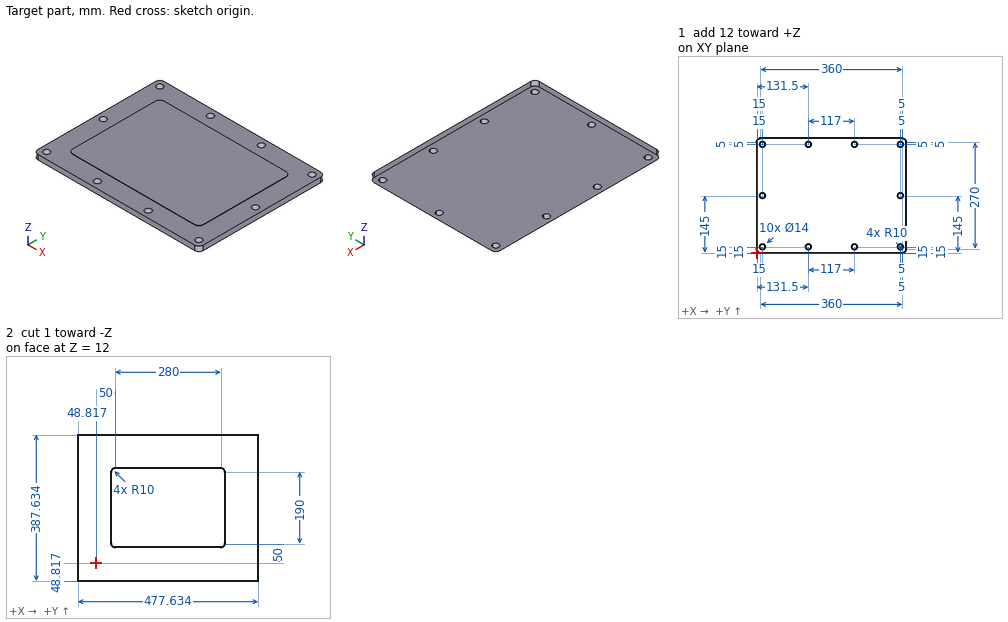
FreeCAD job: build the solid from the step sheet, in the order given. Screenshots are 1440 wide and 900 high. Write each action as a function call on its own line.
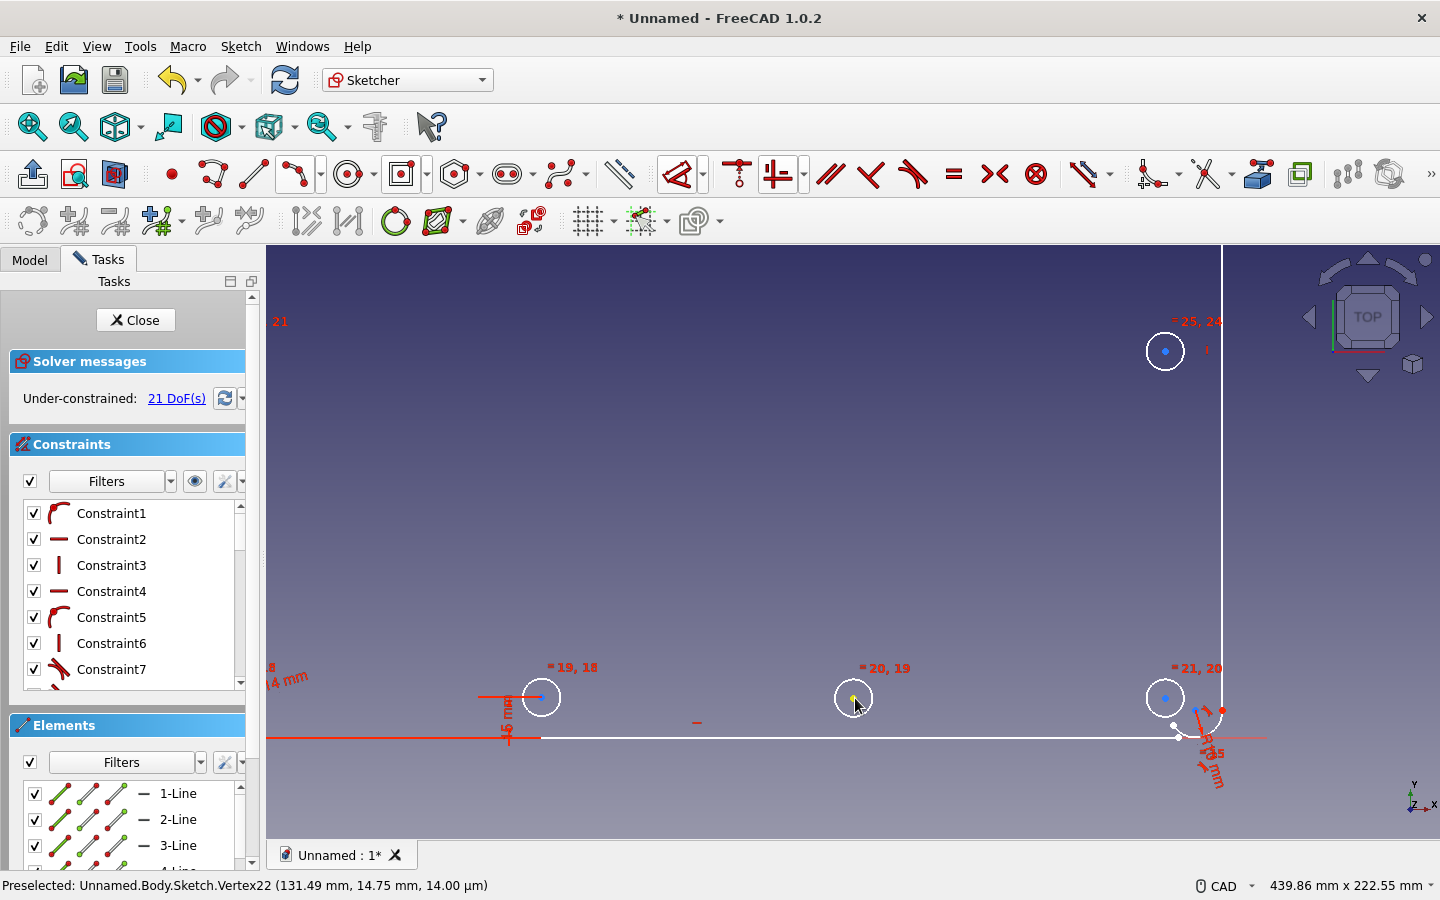
click(854, 698)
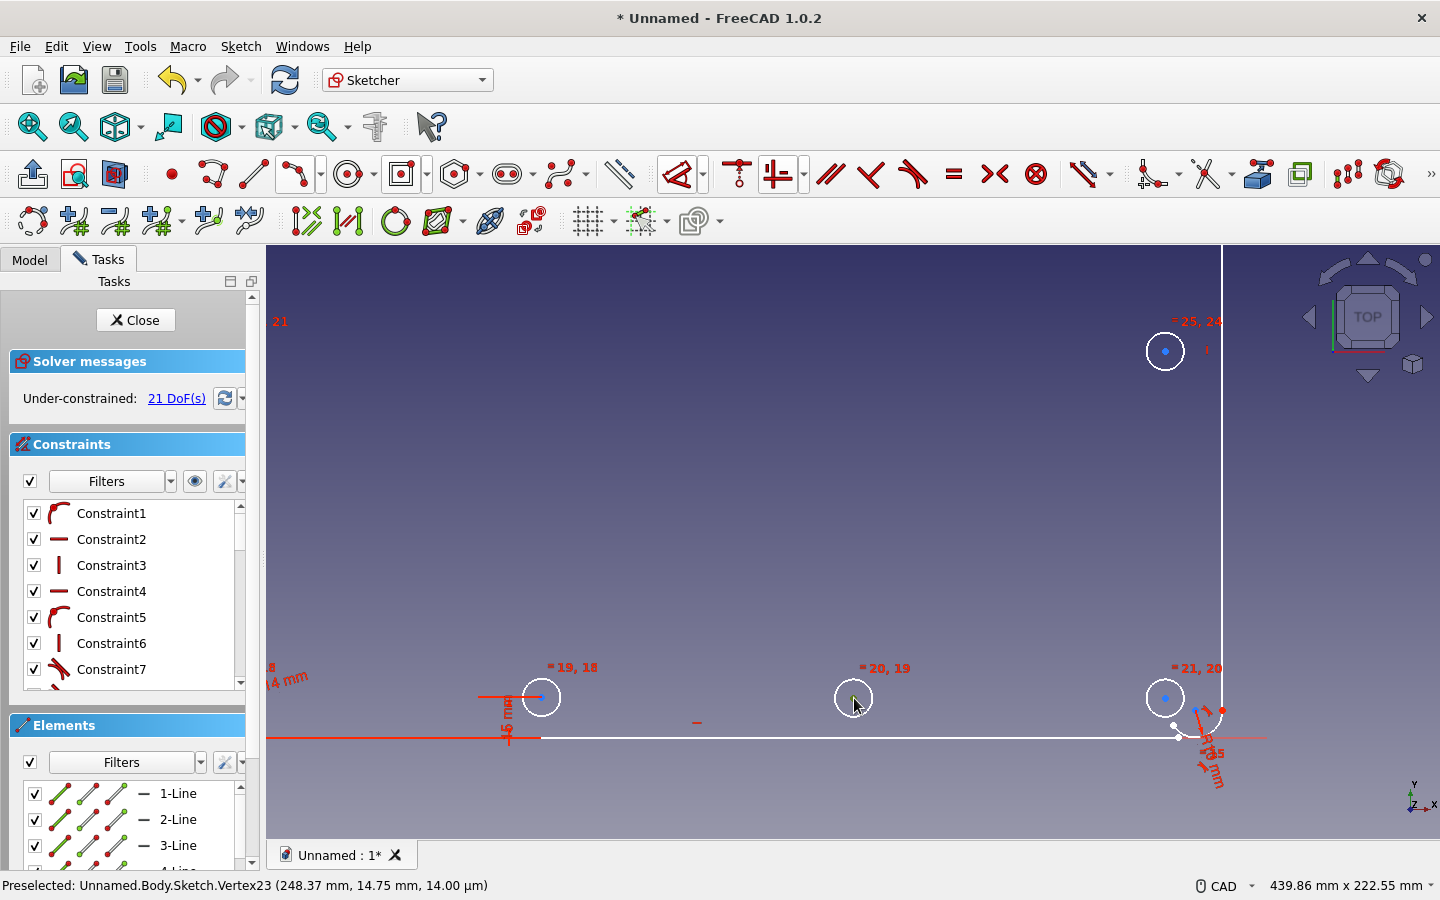
click(702, 174)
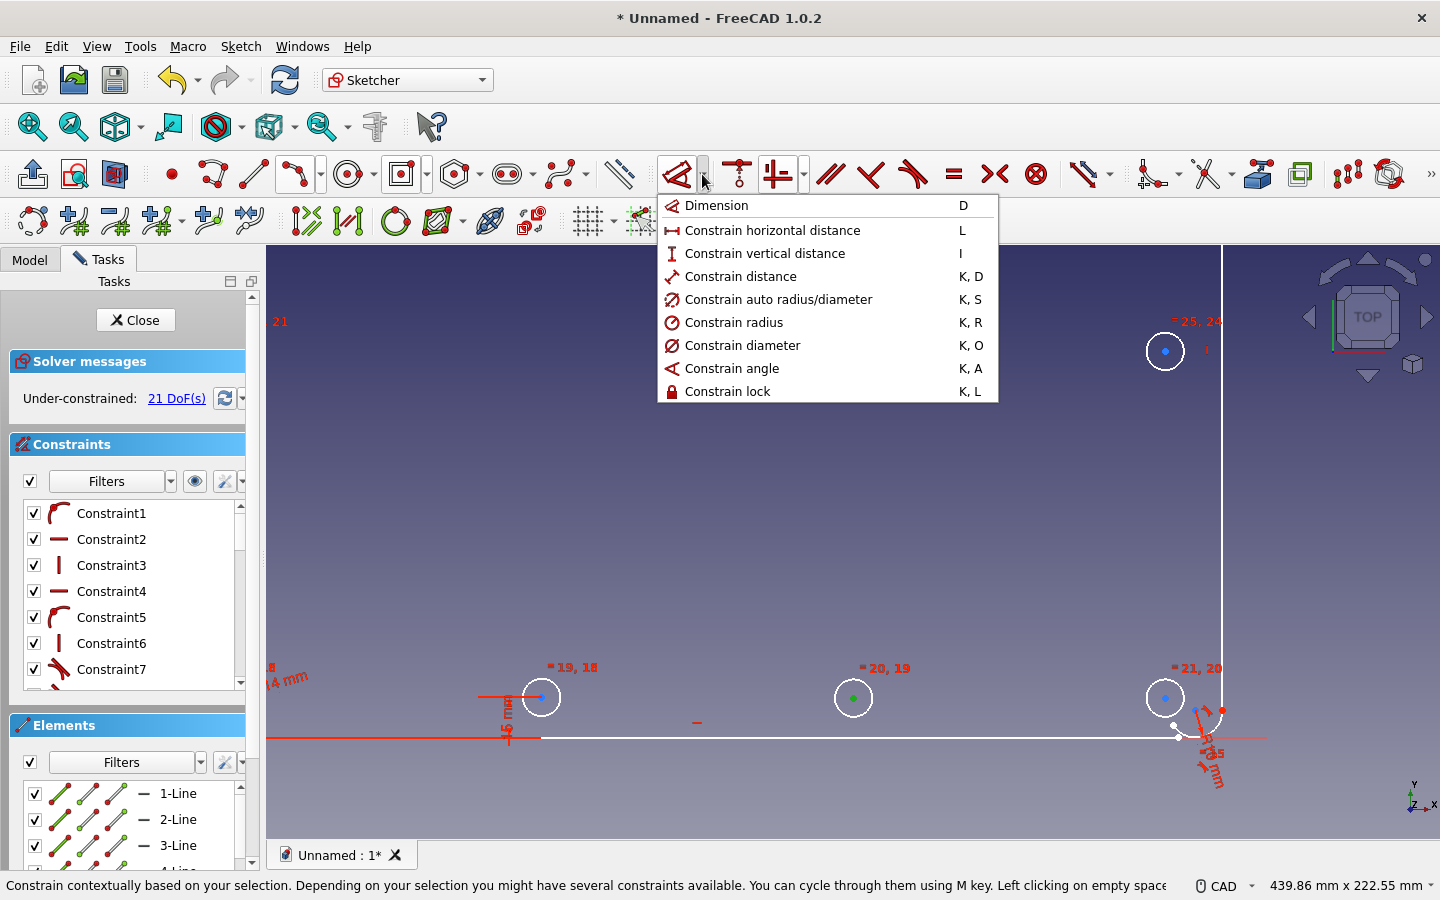
click(828, 254)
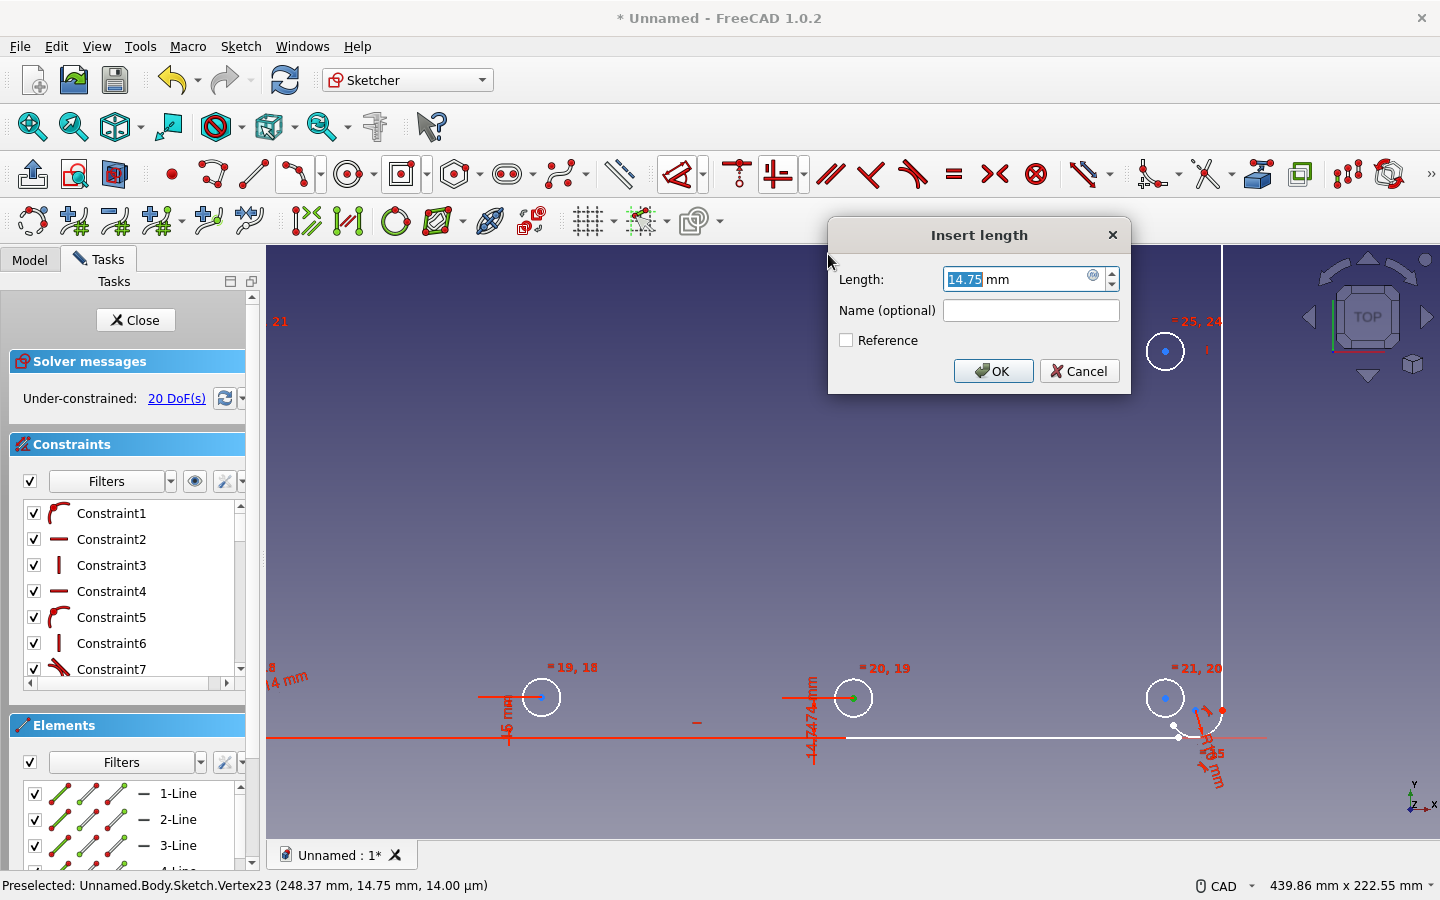
text(15)
key(Return)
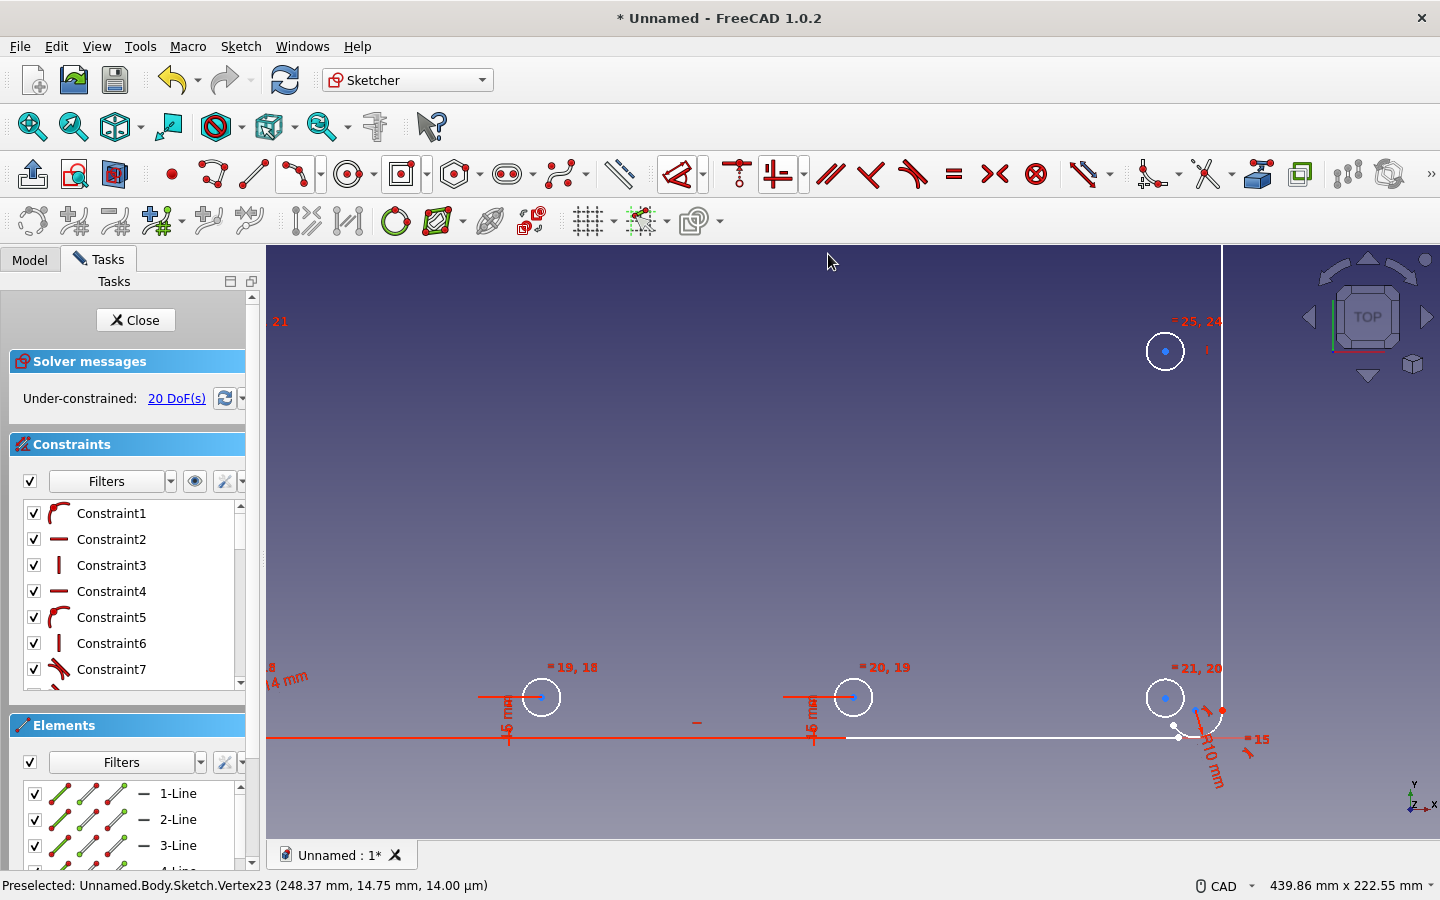
click(1165, 698)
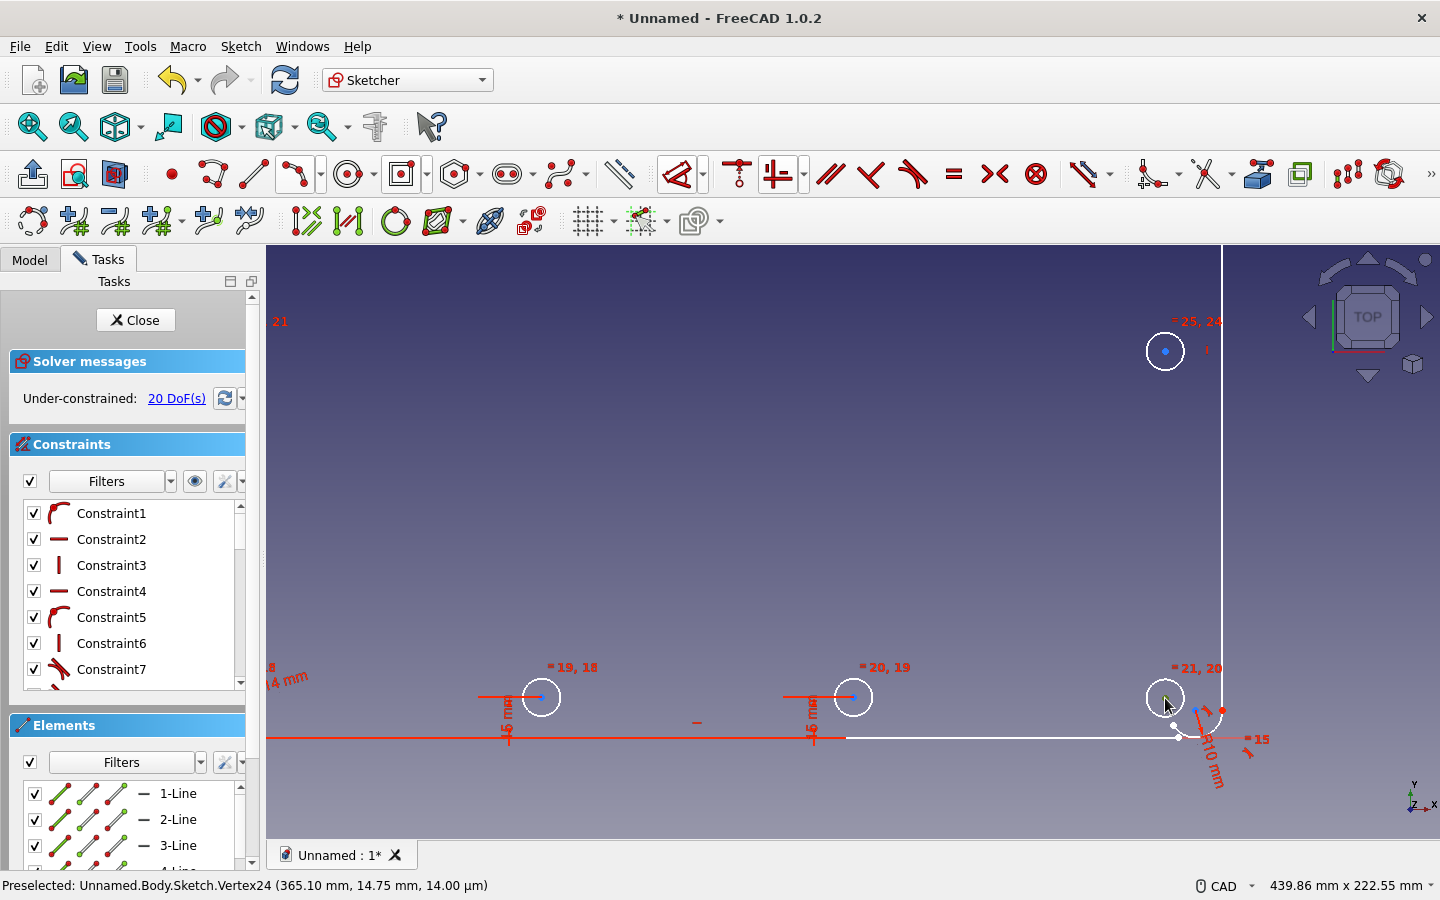
click(702, 174)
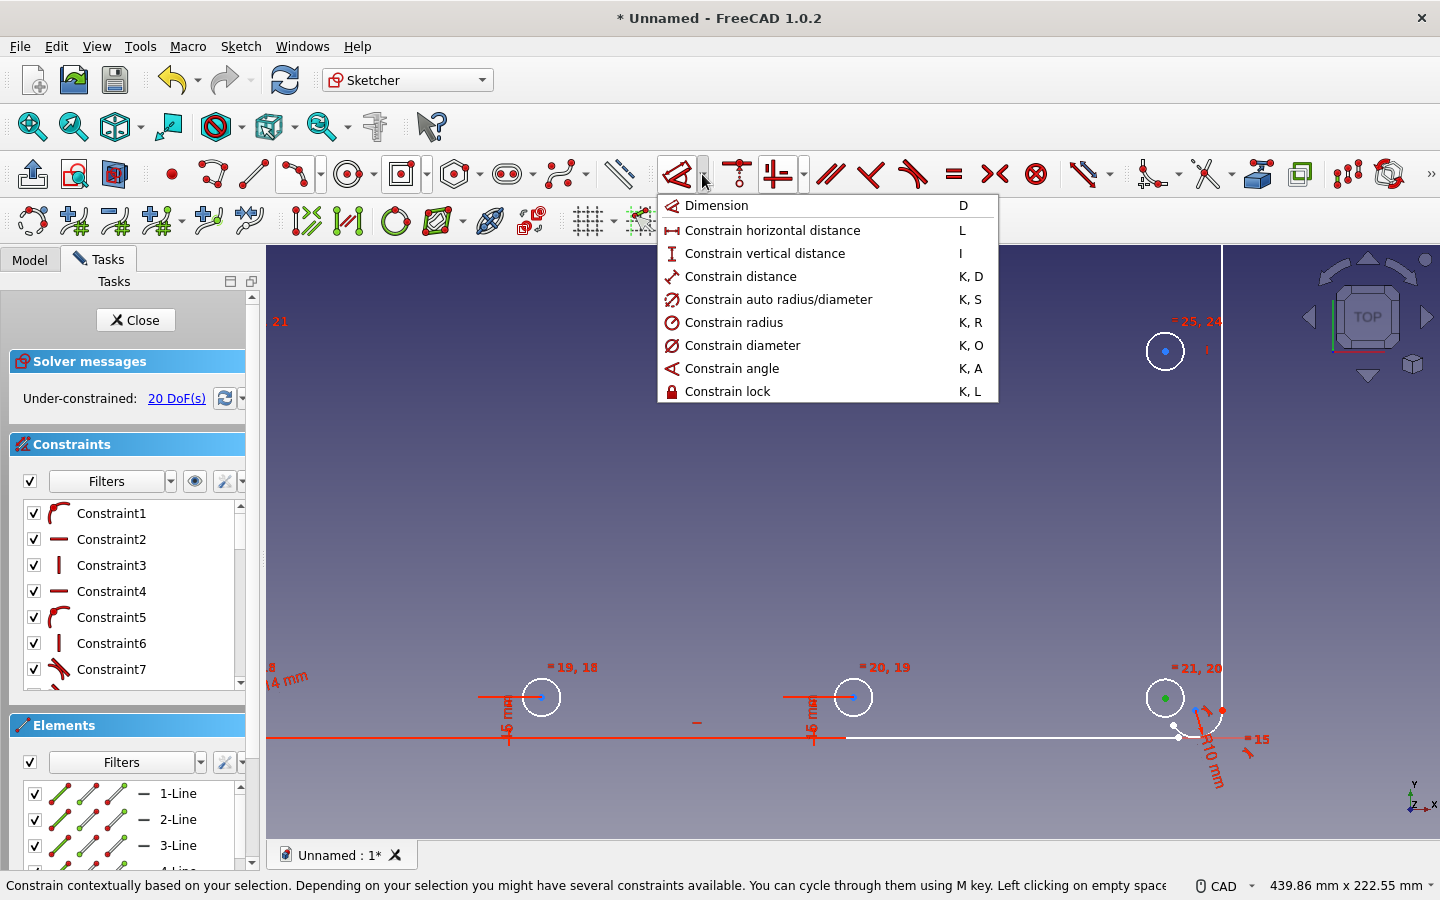
click(828, 254)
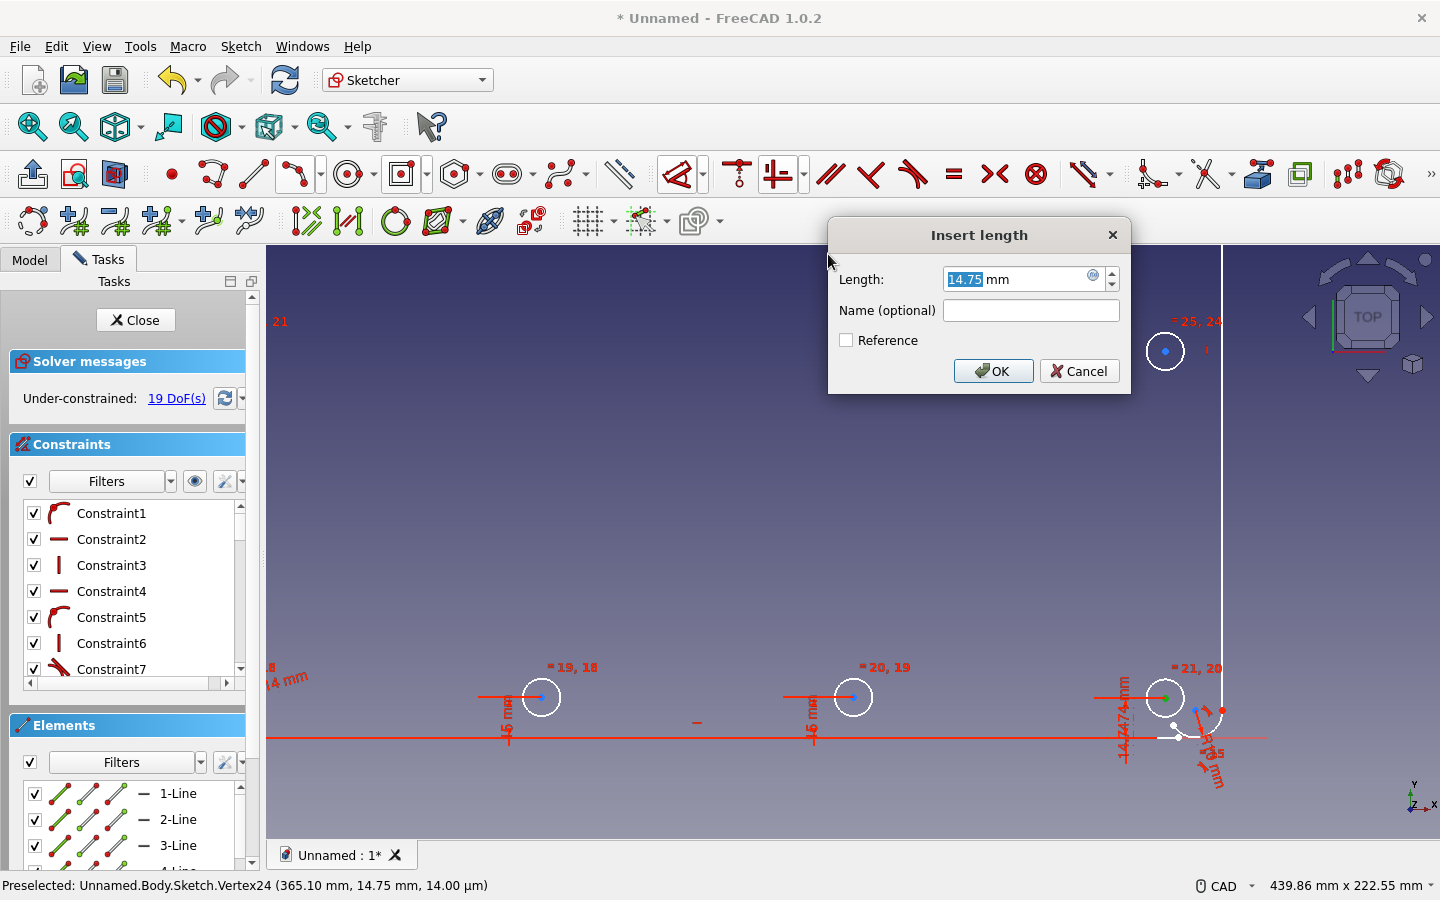
text(15)
key(Return)